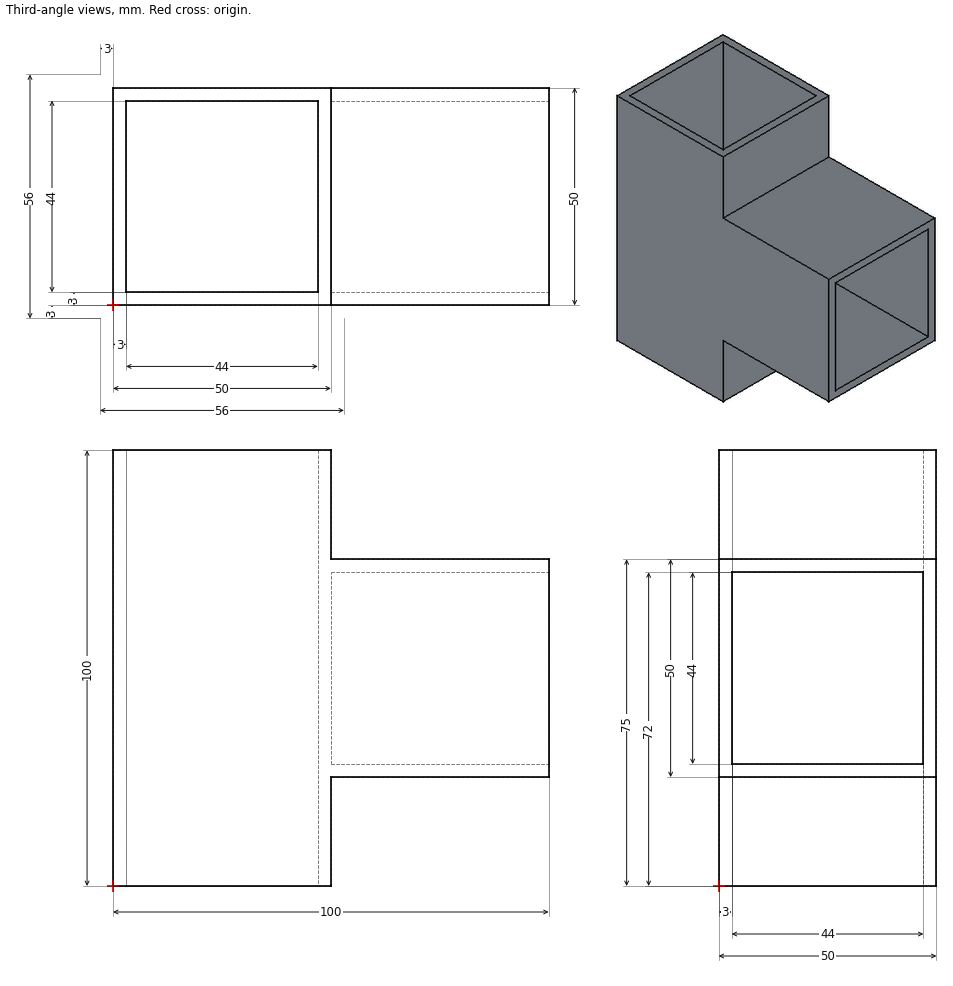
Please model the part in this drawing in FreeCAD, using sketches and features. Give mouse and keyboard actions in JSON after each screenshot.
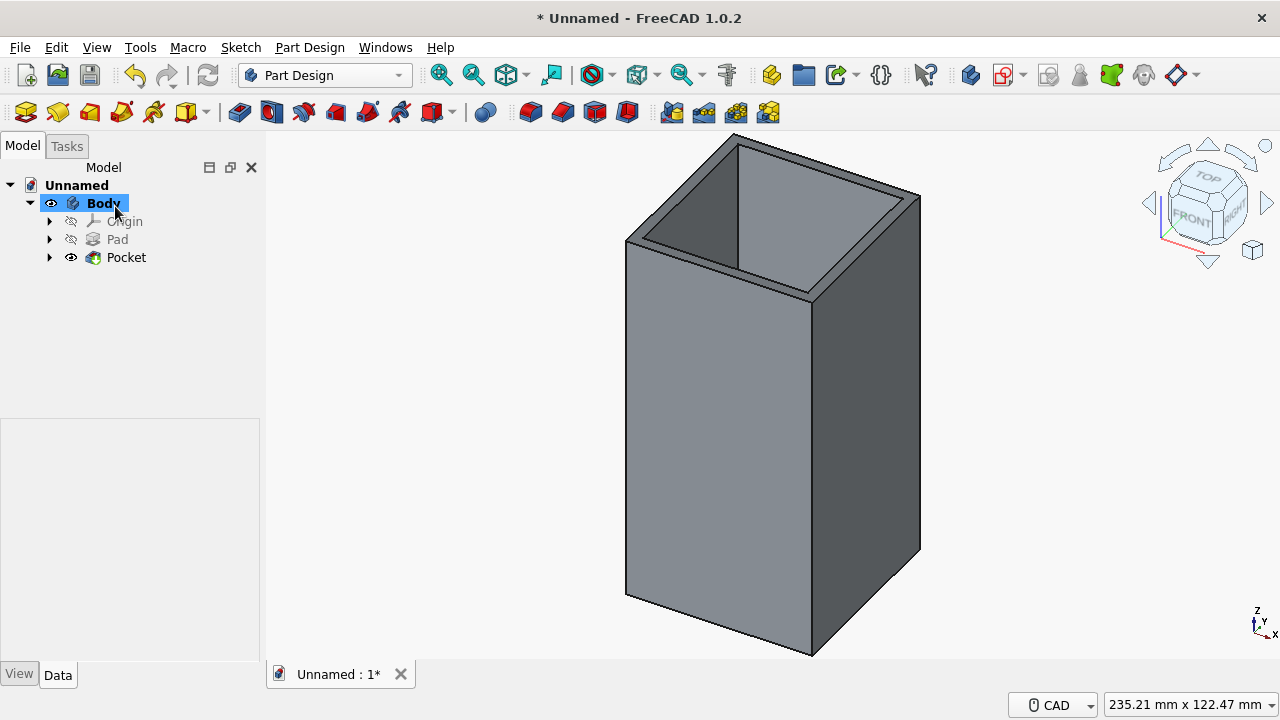
{"action": "left_click", "coordinate": [1004, 76]}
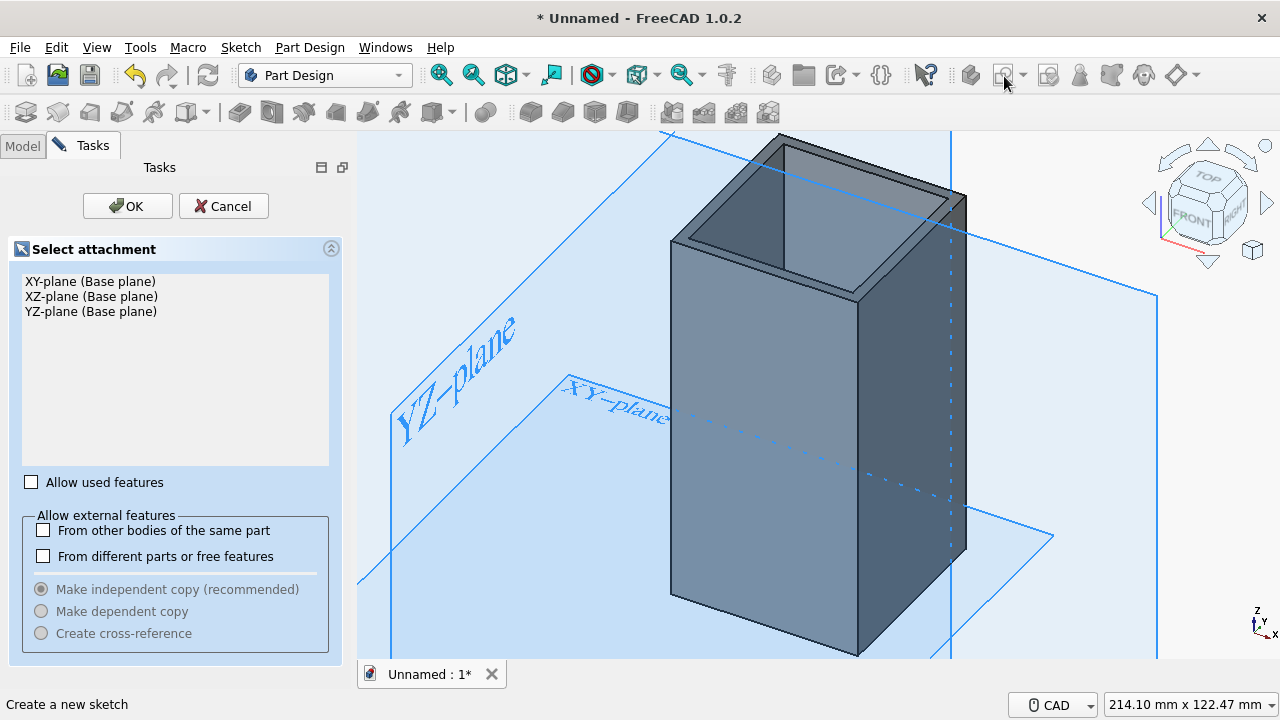
{"action": "left_click", "coordinate": [82, 312]}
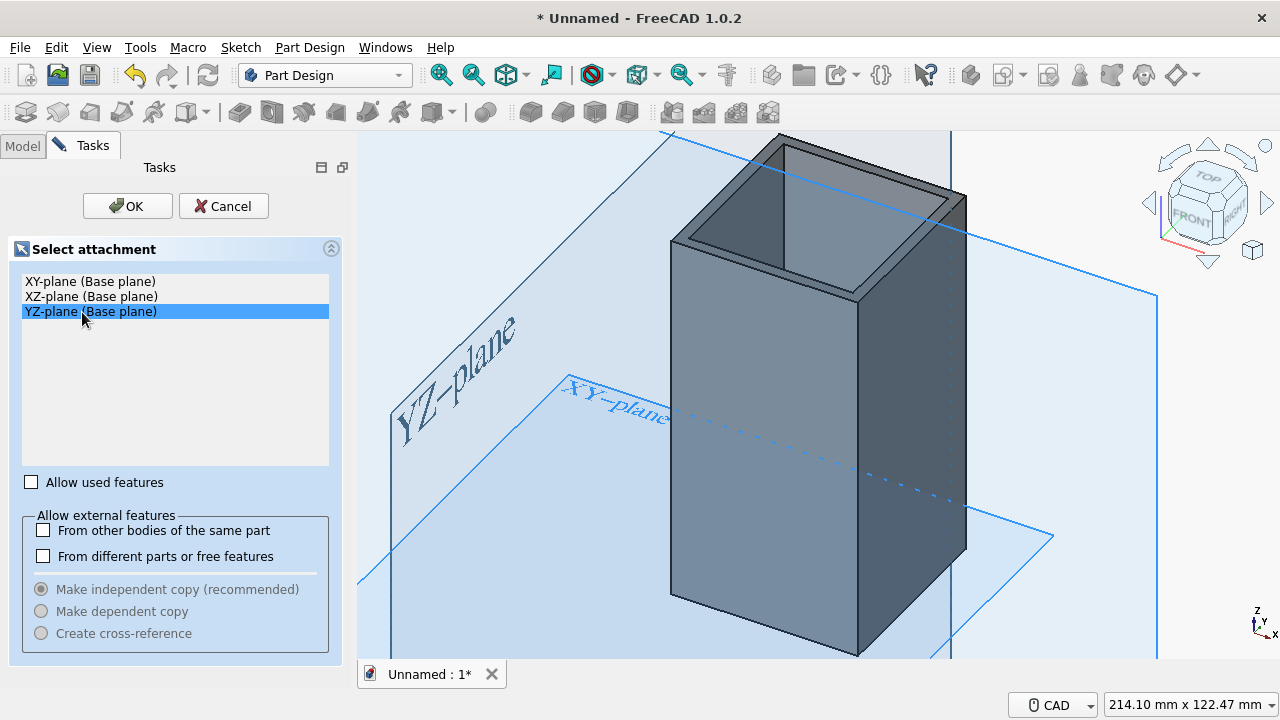
{"action": "left_click", "coordinate": [128, 206]}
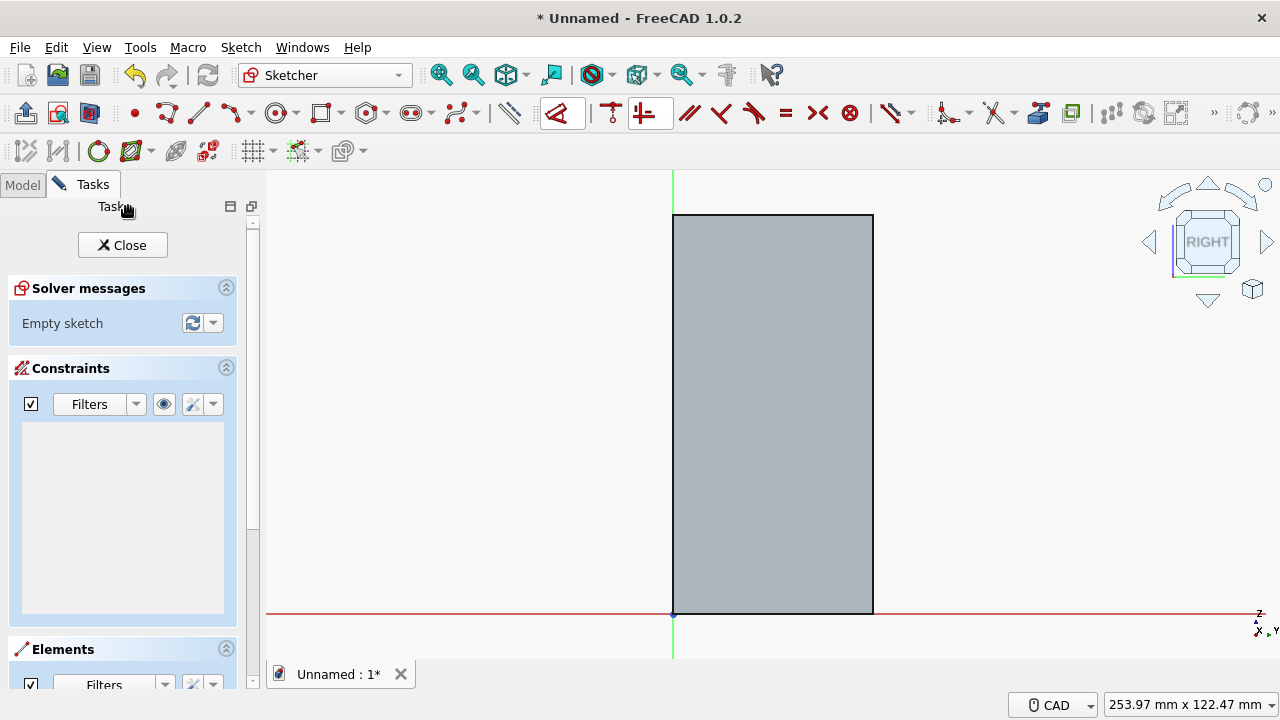
{"action": "left_click", "coordinate": [90, 114]}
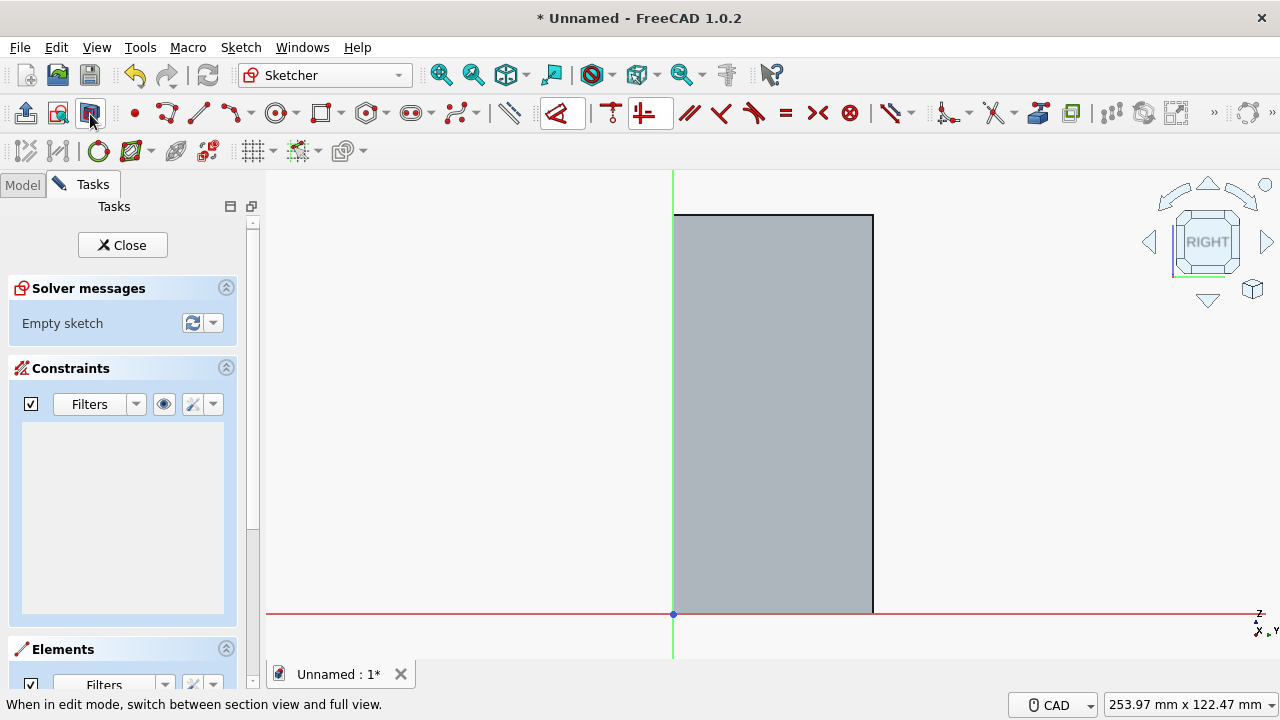
{"action": "scroll", "coordinate": [395, 198], "scroll_direction": "down", "scroll_amount": 1}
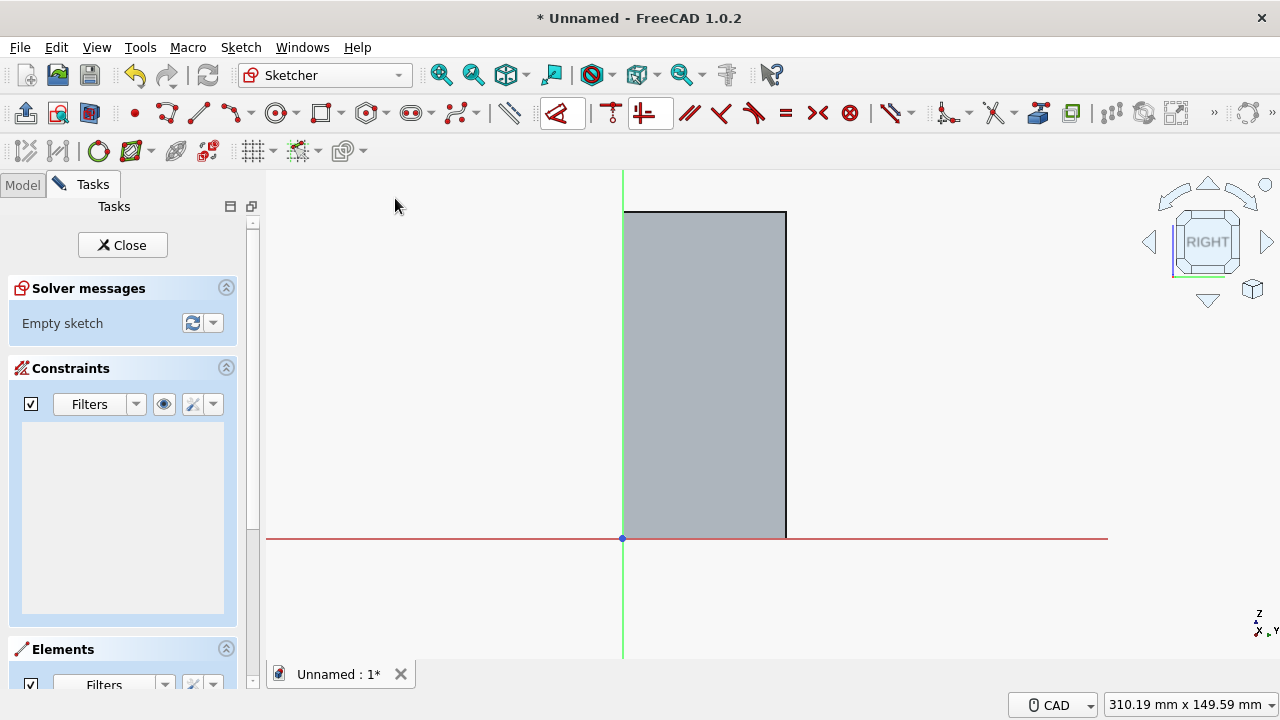
{"action": "key", "text": "g r"}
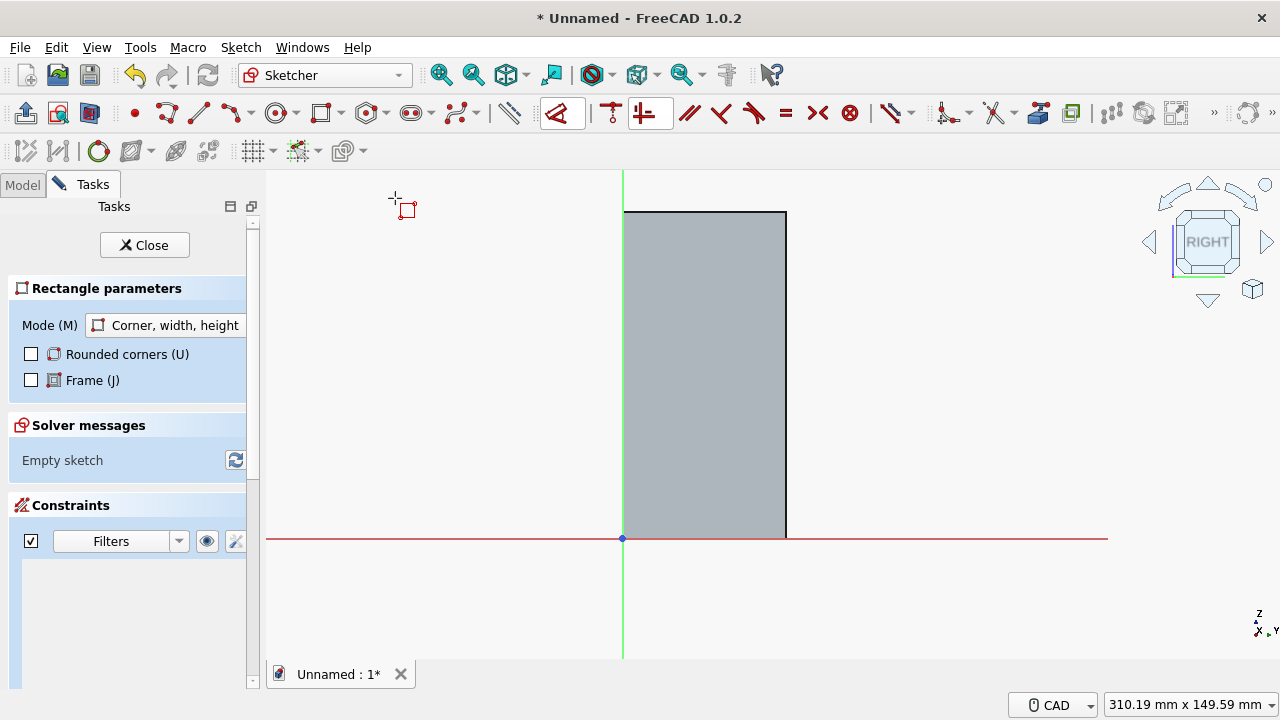
{"action": "left_click", "coordinate": [623, 294]}
{"action": "left_click", "coordinate": [786, 457]}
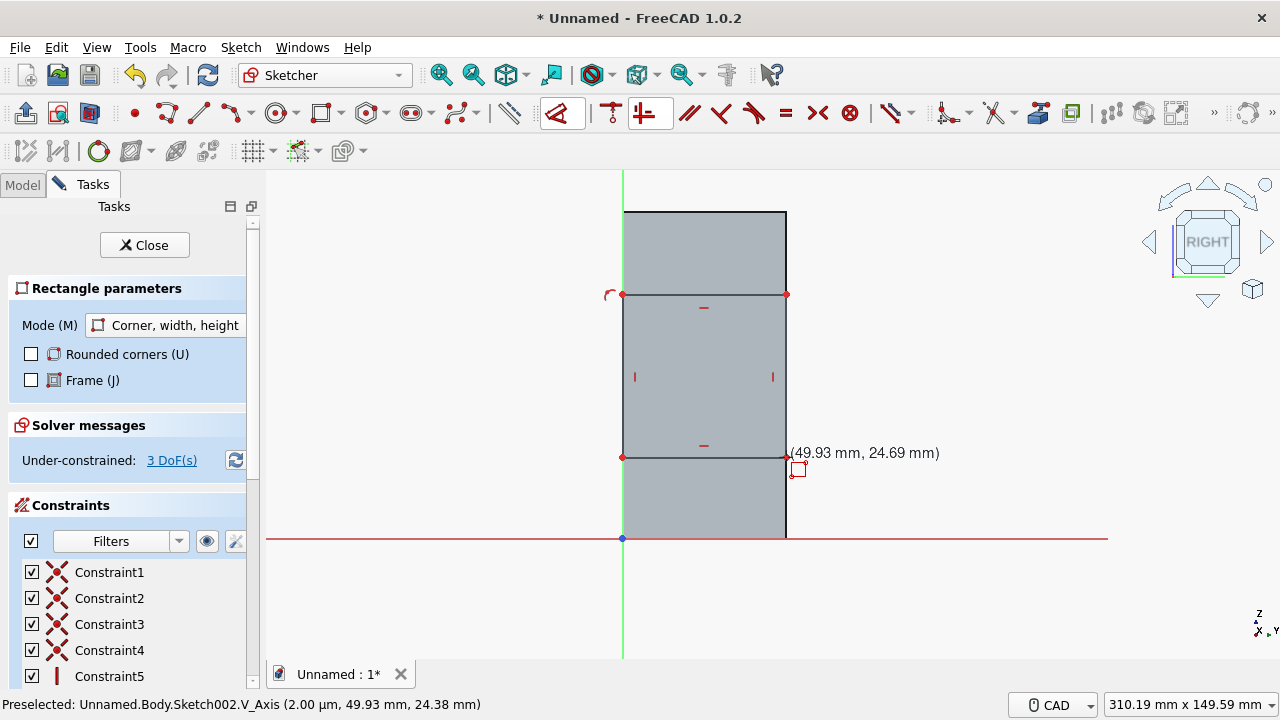
{"action": "scroll", "coordinate": [633, 303], "scroll_direction": "up", "scroll_amount": 3}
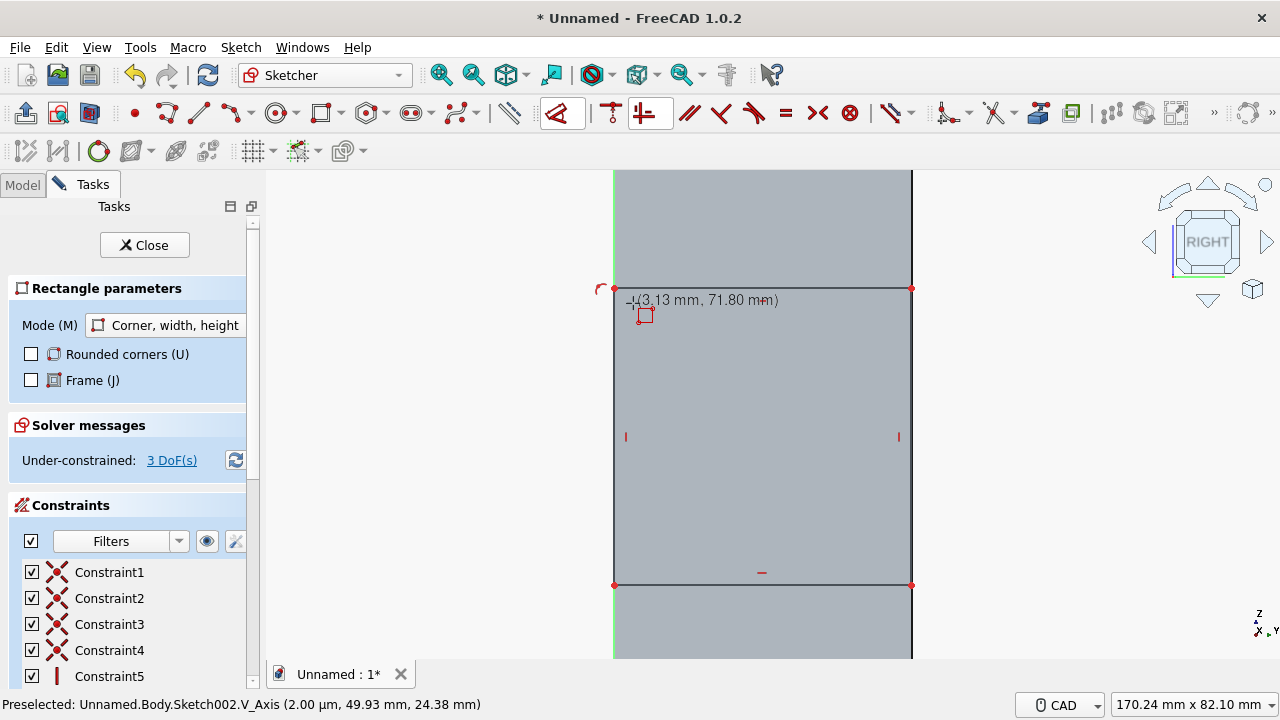
{"action": "left_click", "coordinate": [632, 303]}
{"action": "left_click", "coordinate": [894, 565]}
{"action": "key", "text": "Escape"}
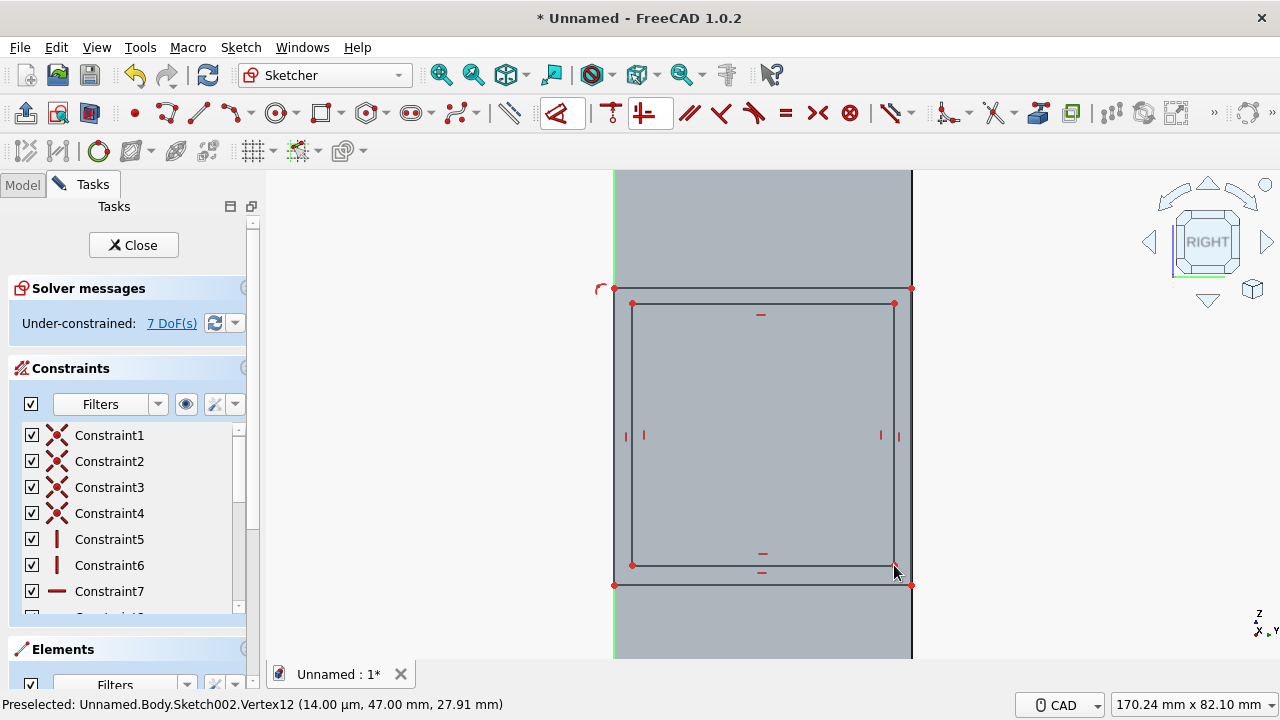
{"action": "left_click", "coordinate": [614, 377]}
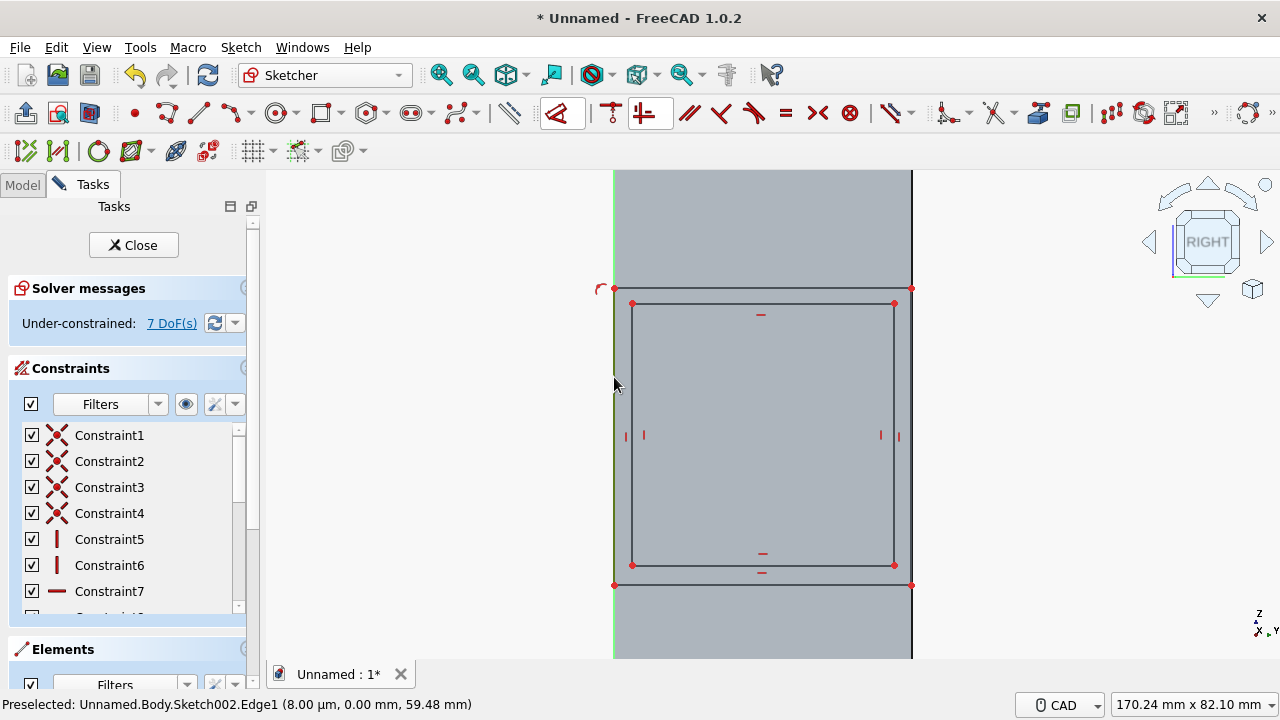
{"action": "key", "text": "i"}